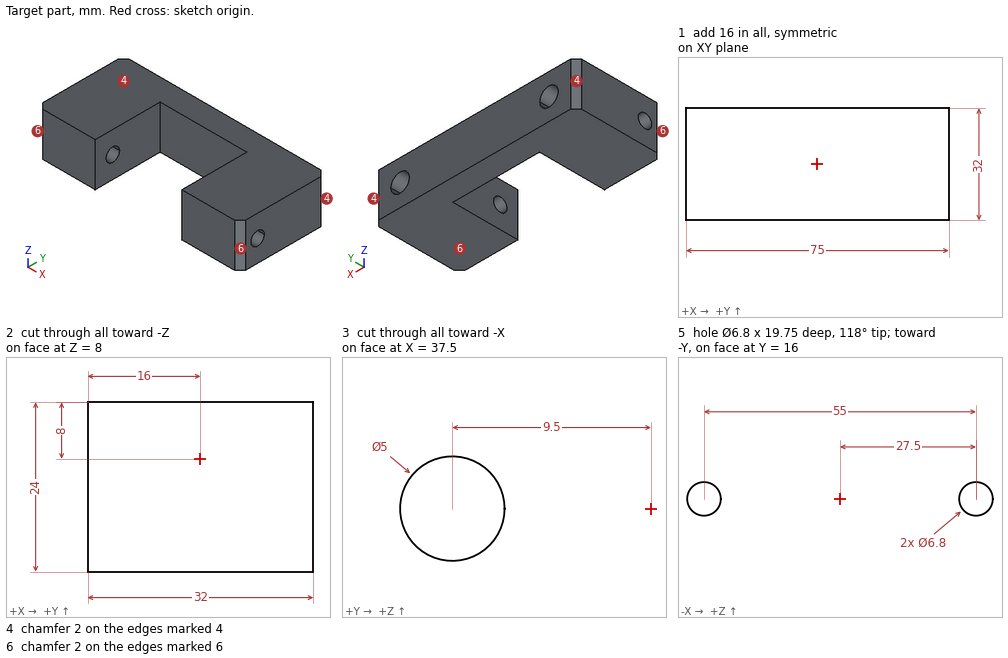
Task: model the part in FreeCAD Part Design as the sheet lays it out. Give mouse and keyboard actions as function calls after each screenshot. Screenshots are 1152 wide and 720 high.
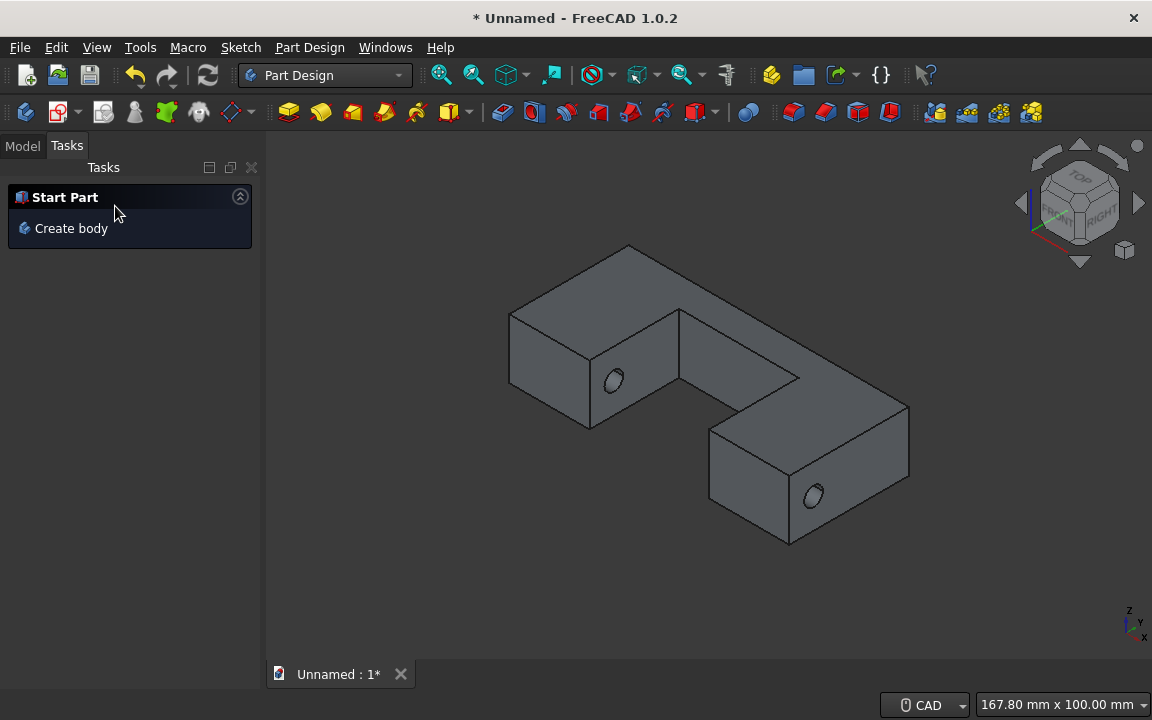
key(2)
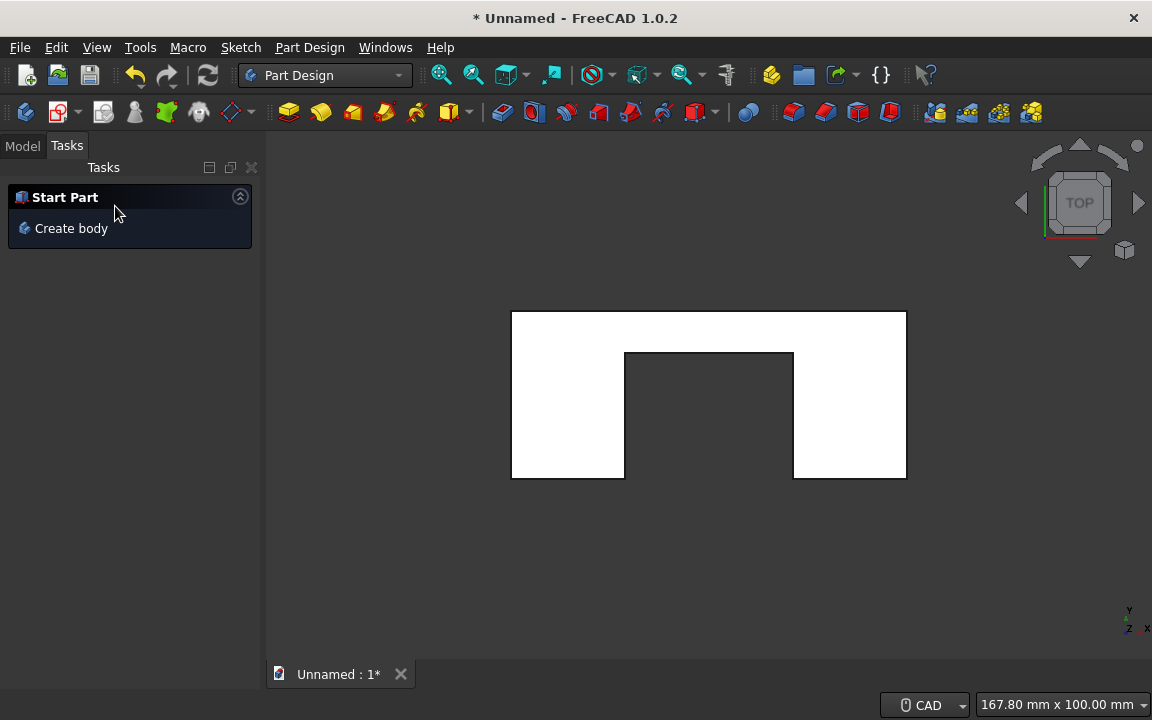
key(v)
key(f)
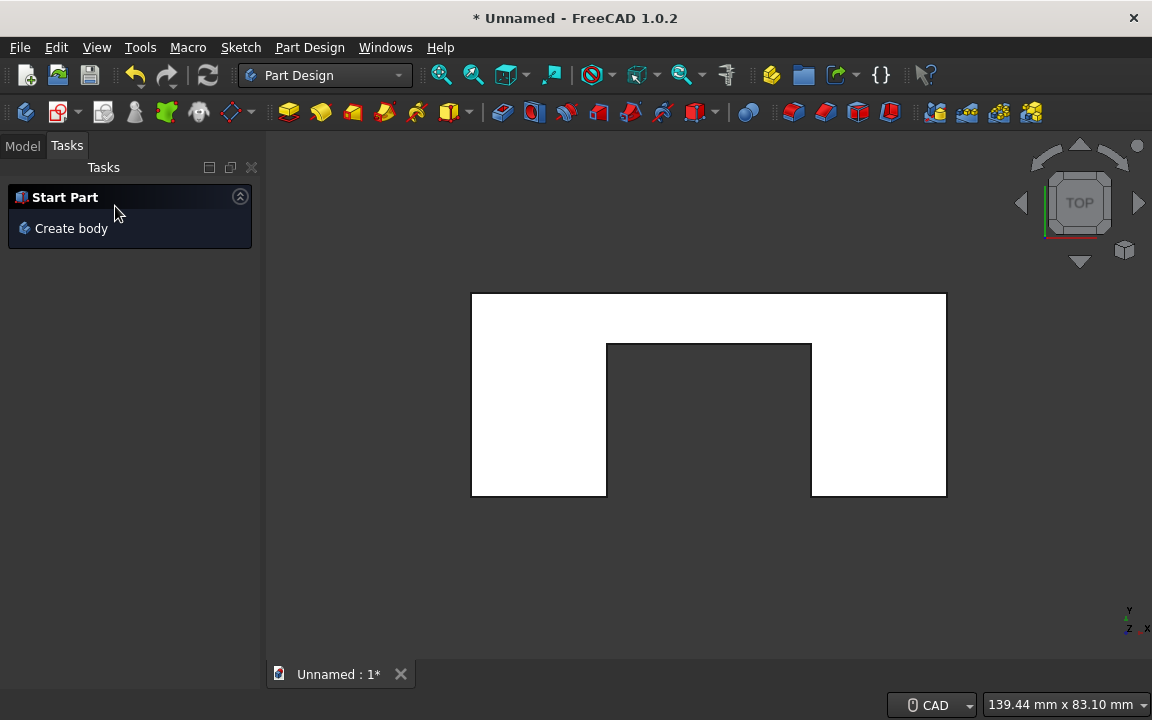
key(1)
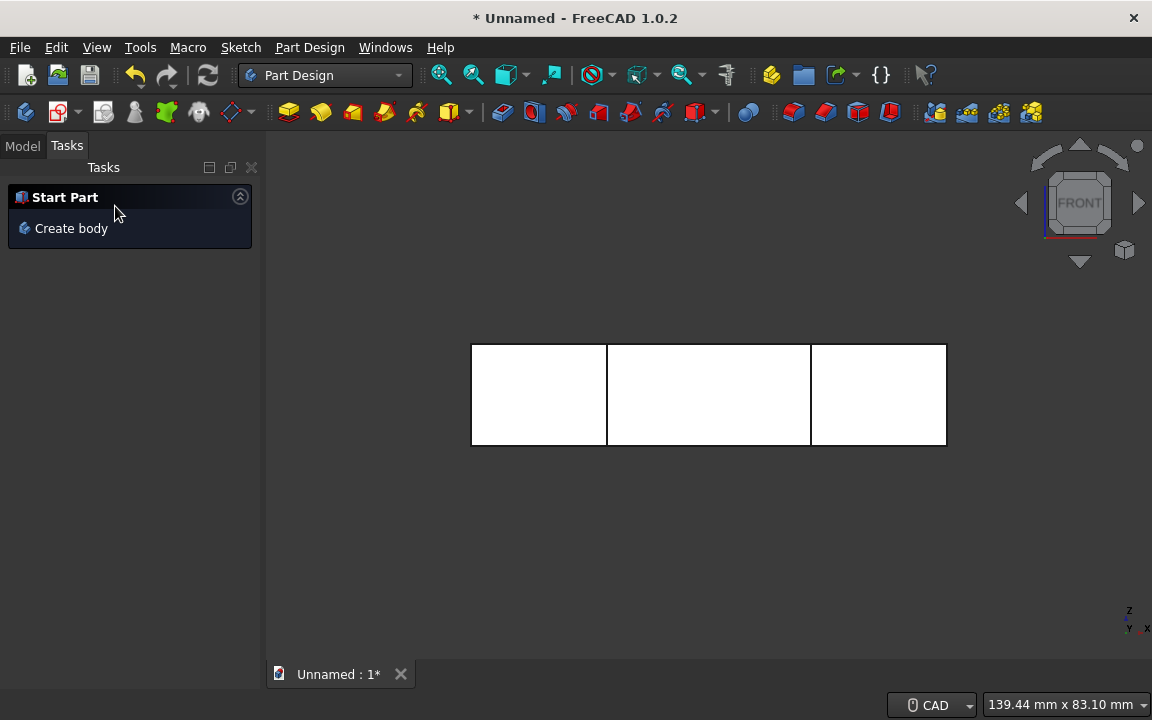
key(3)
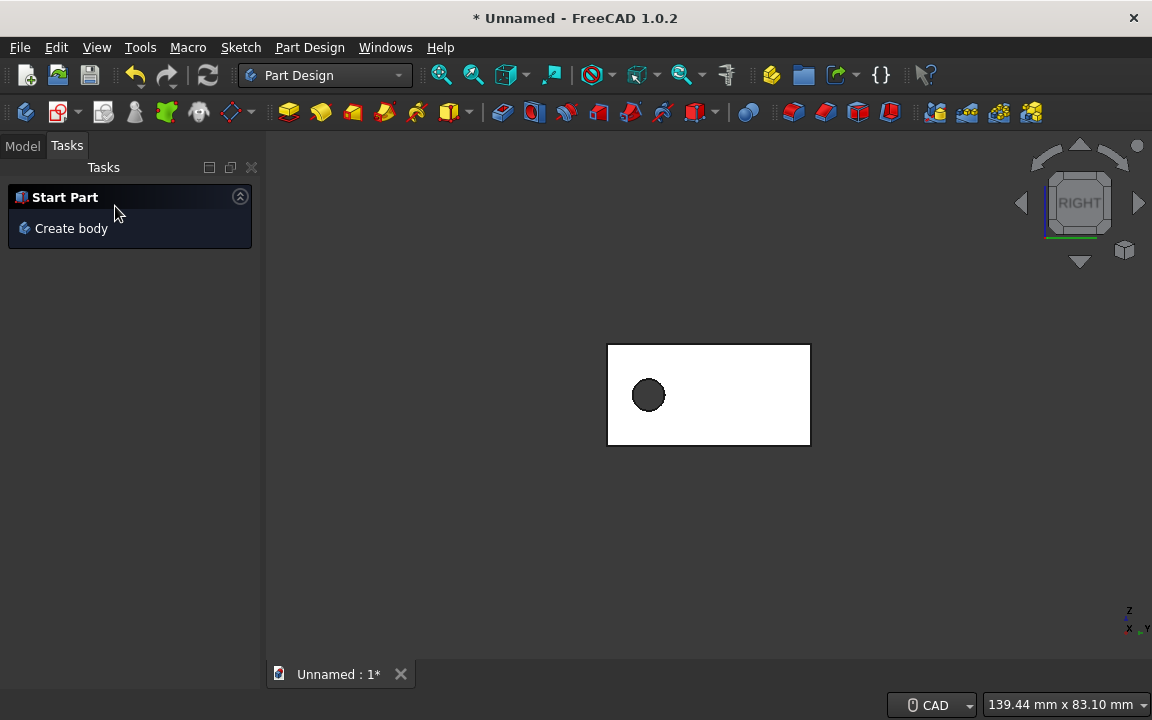
click(442, 76)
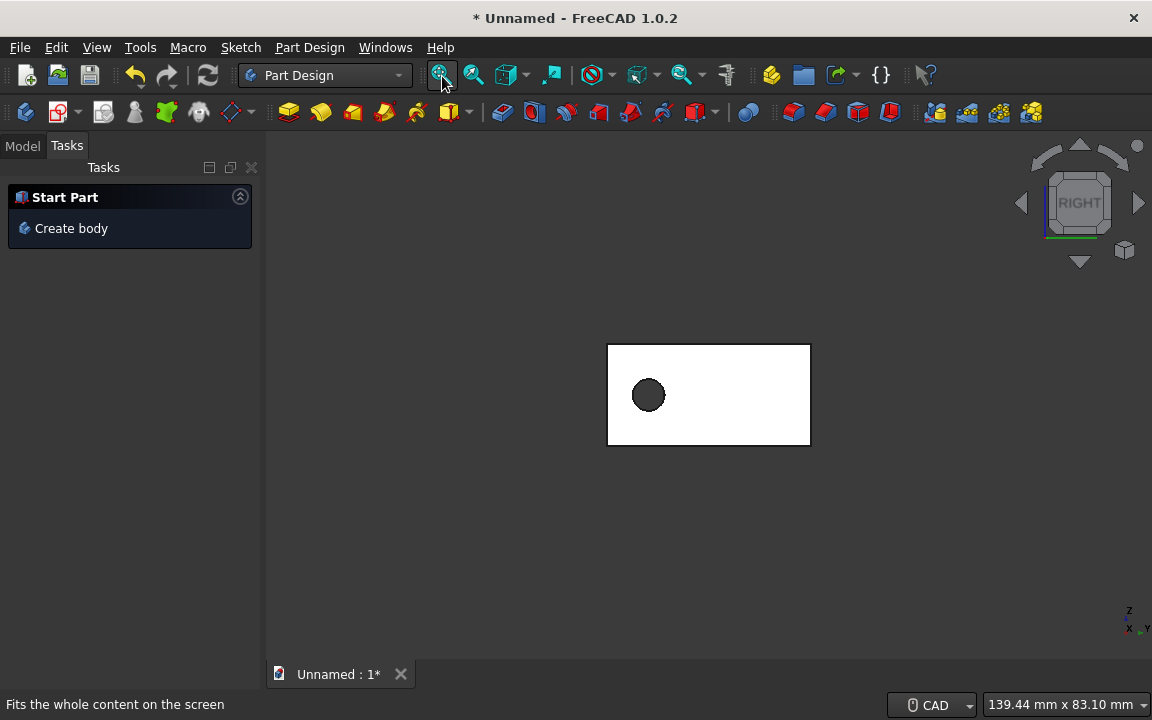
click(811, 394)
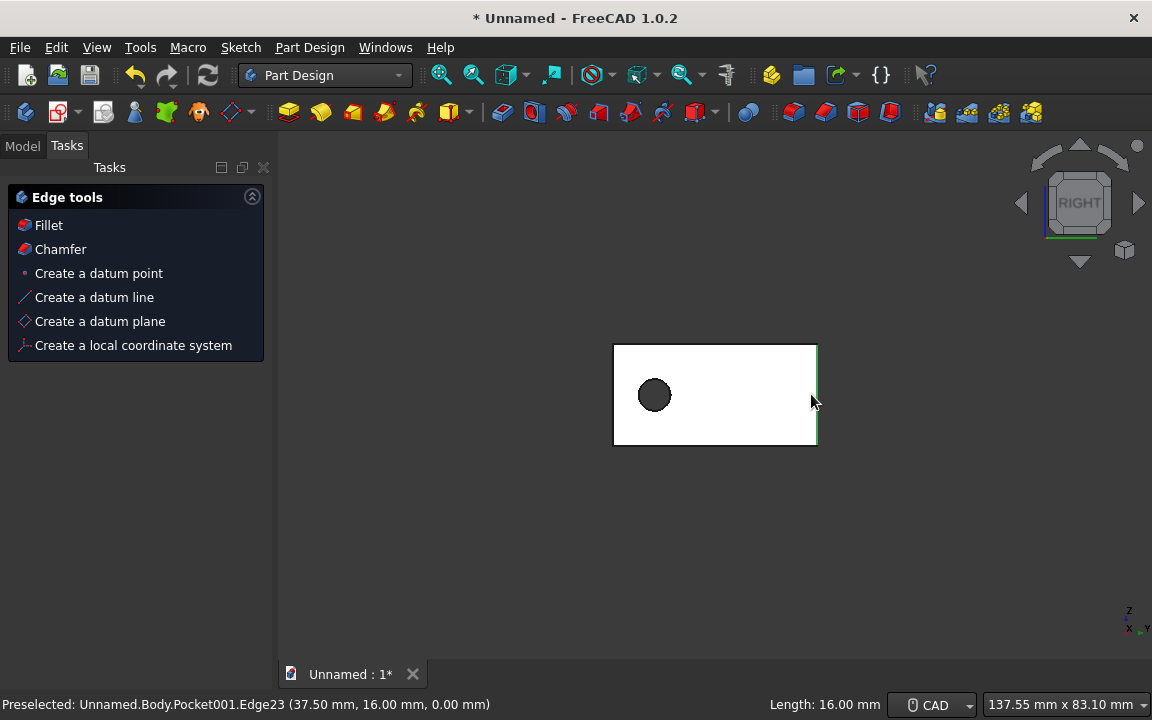
key(5)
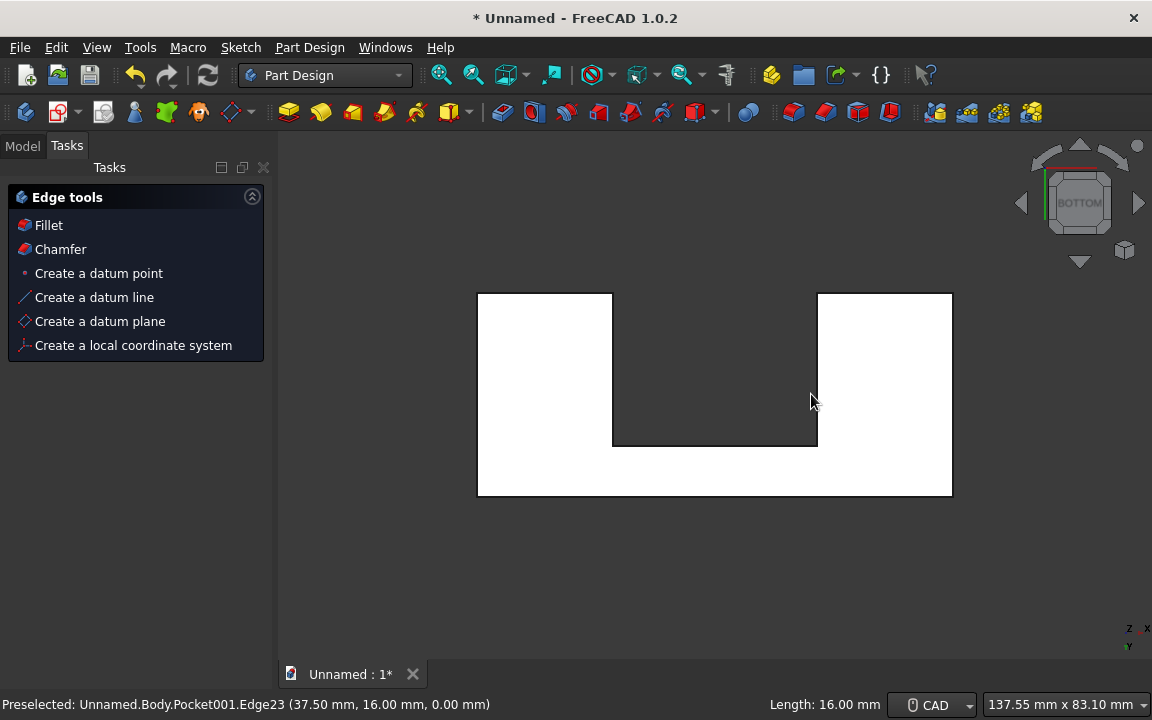
key(4)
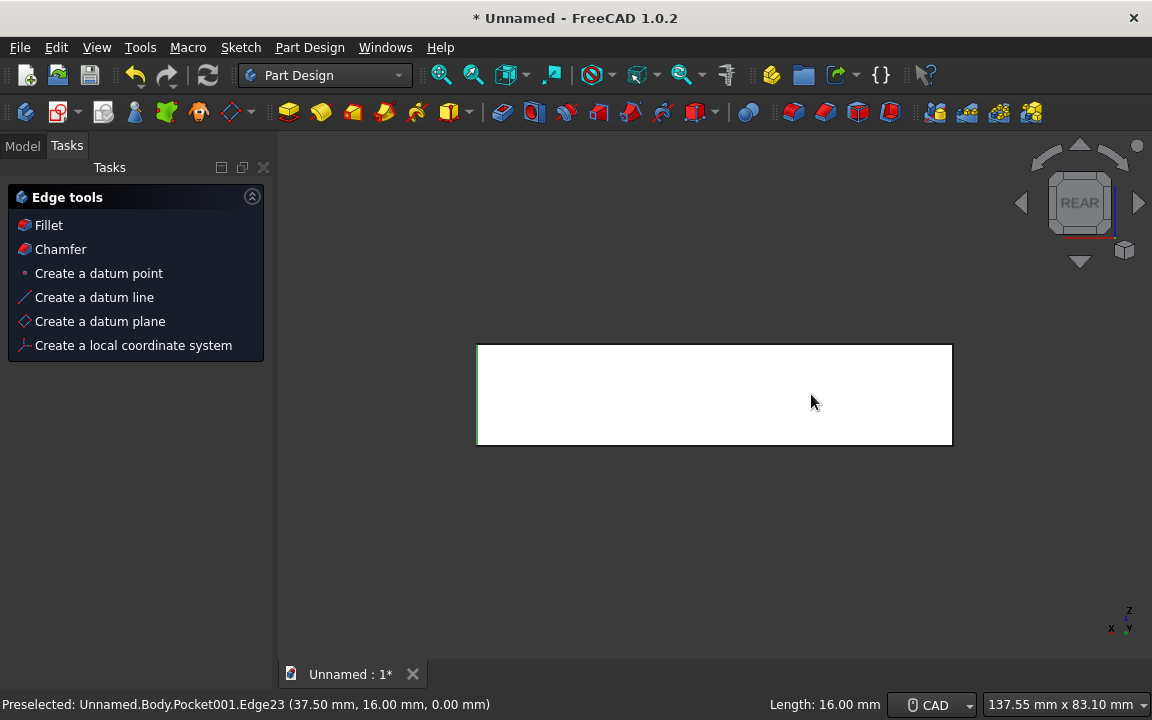
click(953, 394, ctrl)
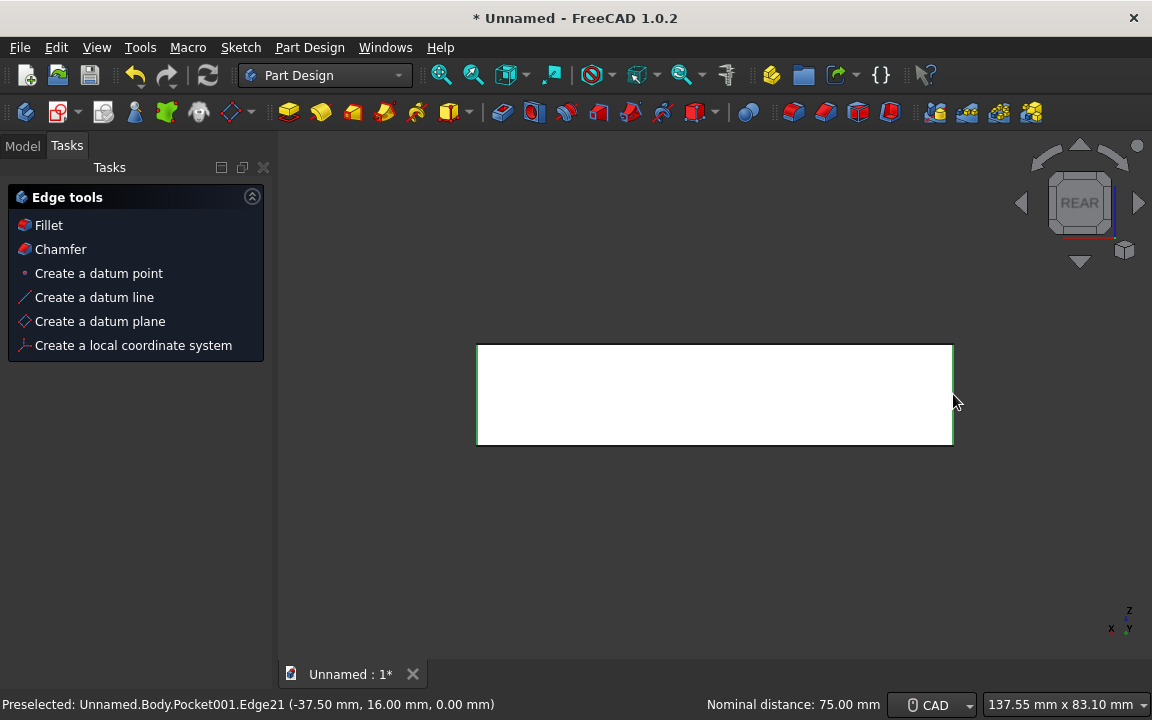
click(826, 112)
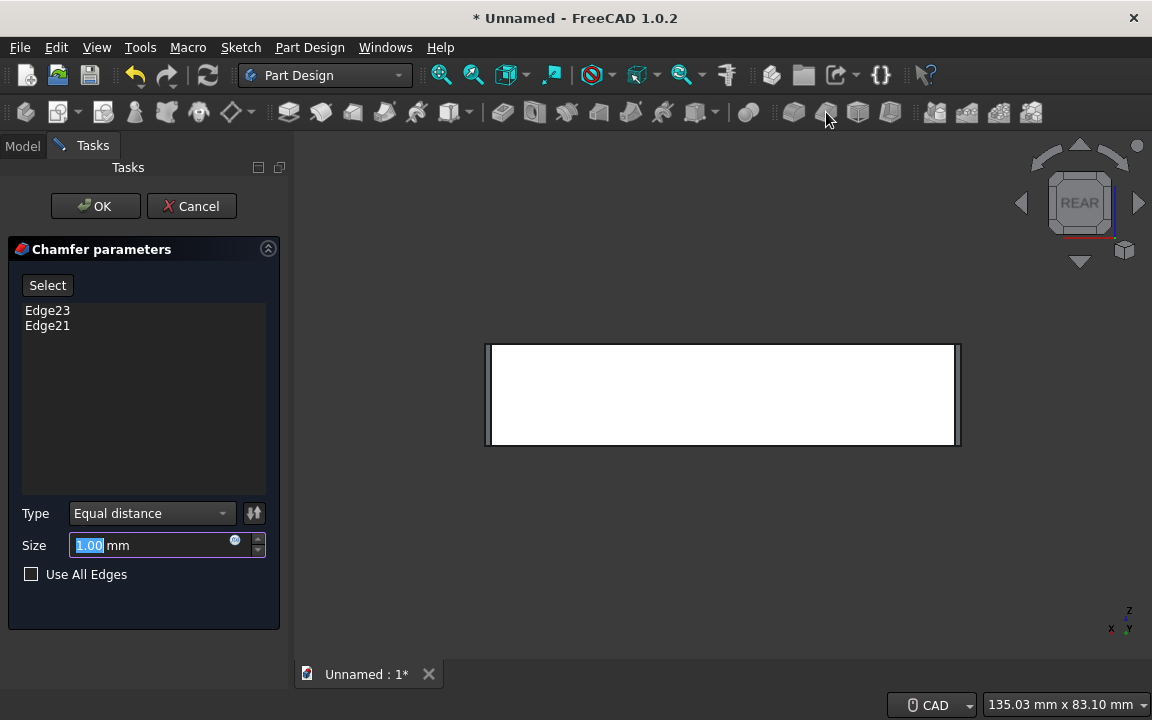
text(2)
key(Tab)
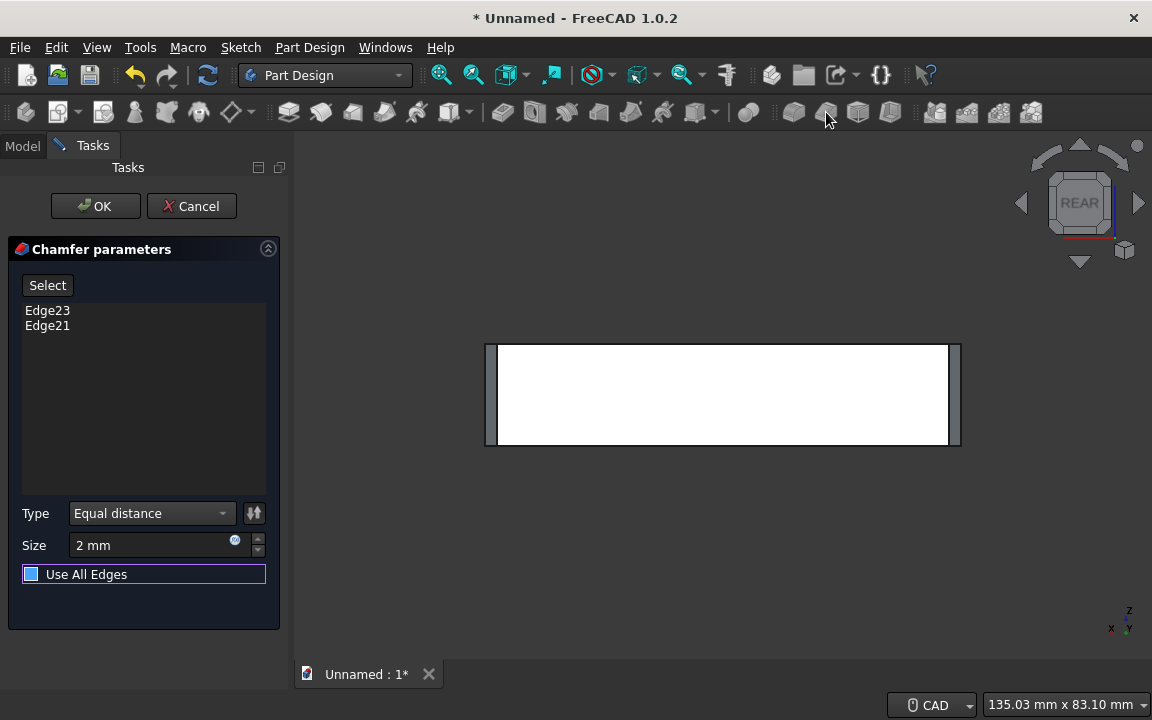
click(96, 206)